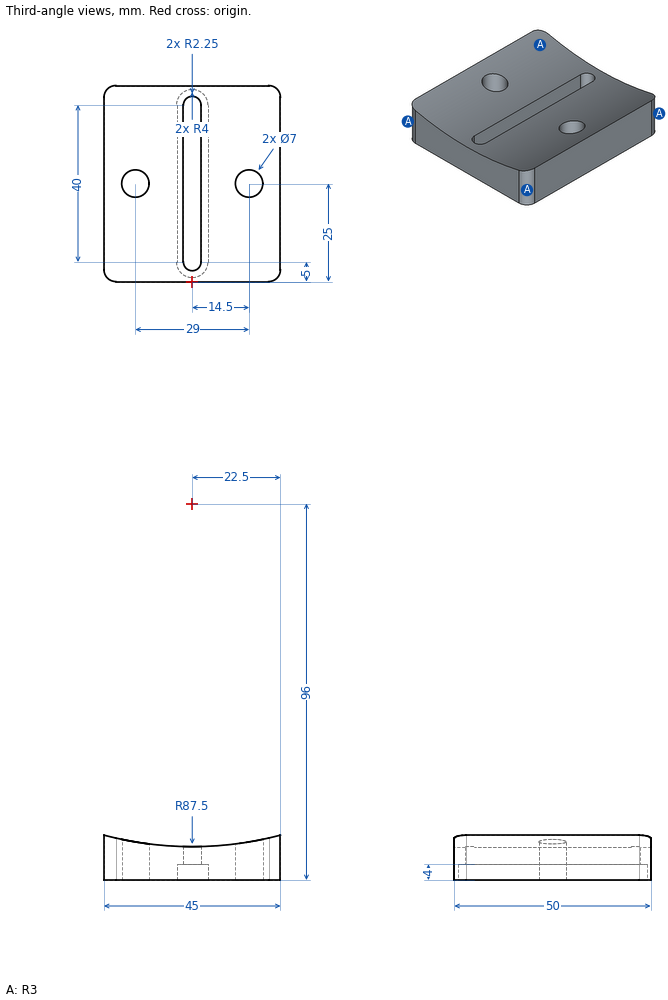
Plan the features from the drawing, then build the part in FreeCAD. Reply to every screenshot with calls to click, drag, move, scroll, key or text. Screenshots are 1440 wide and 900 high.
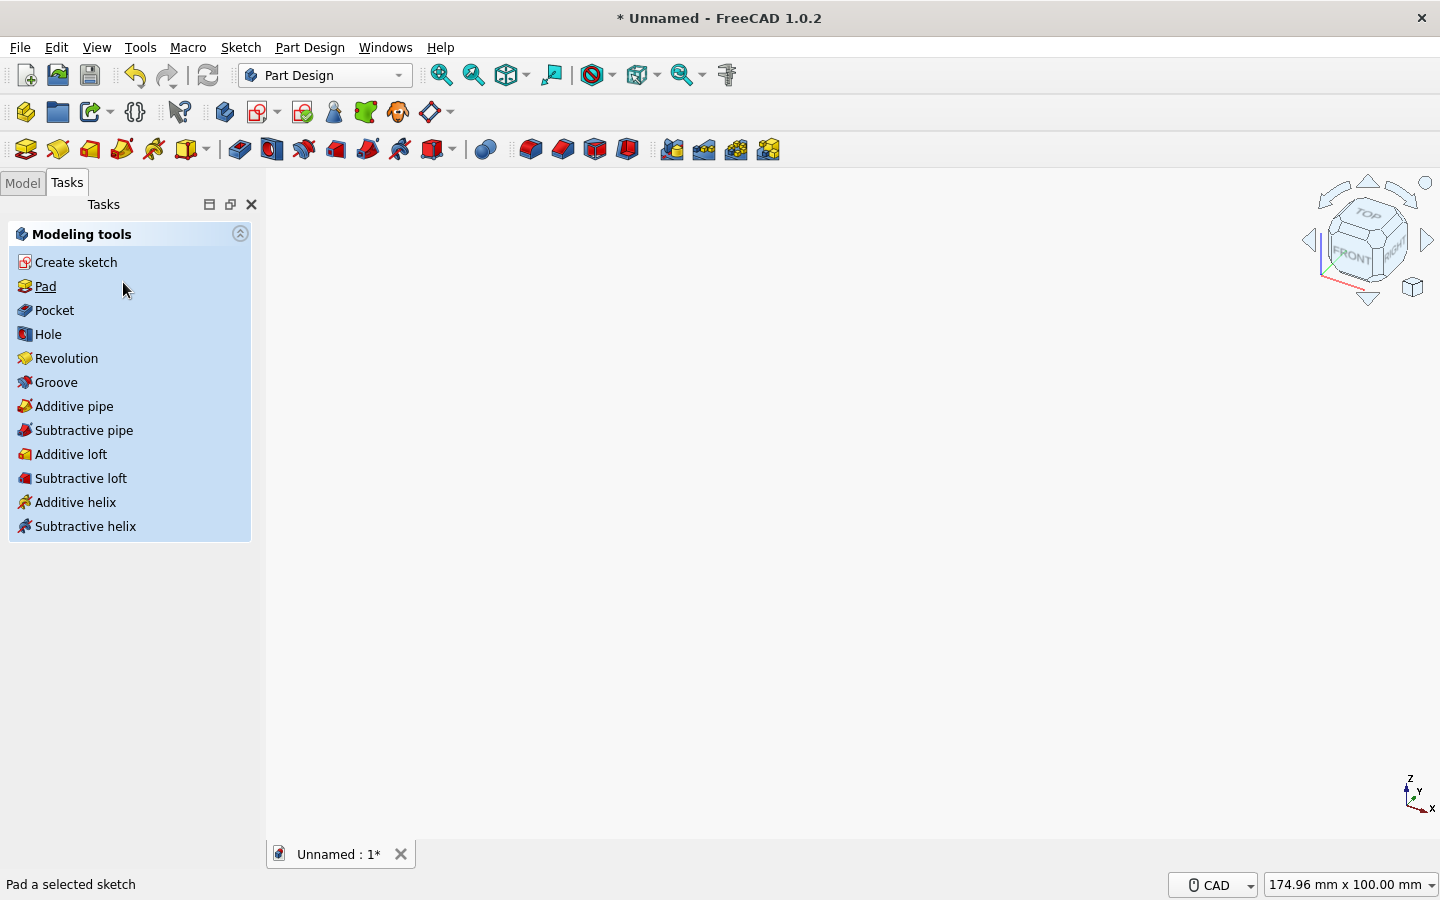
click(26, 150)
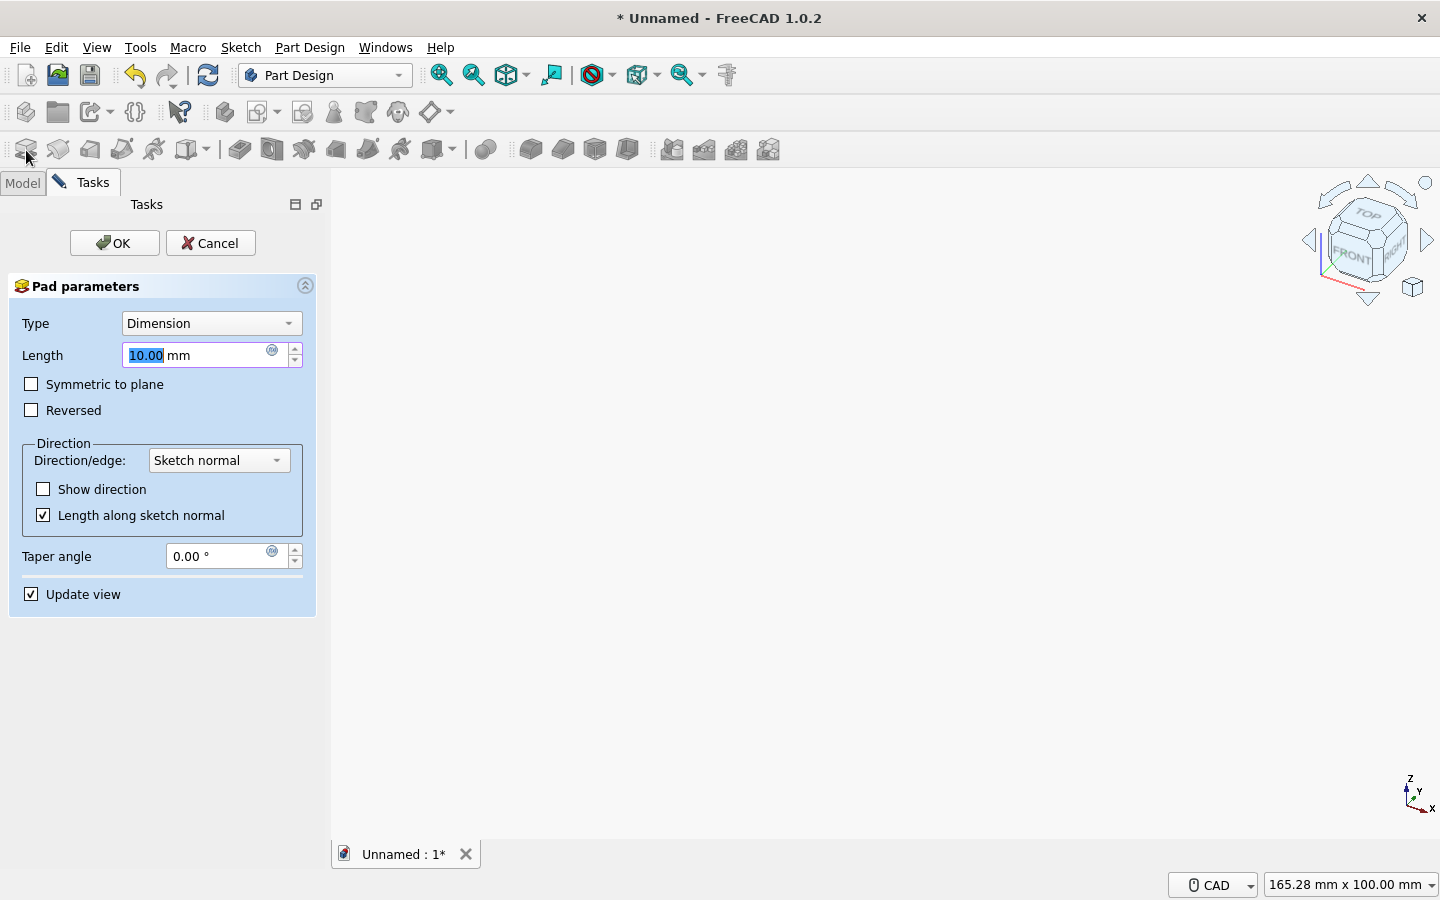
text(50)
key(Tab)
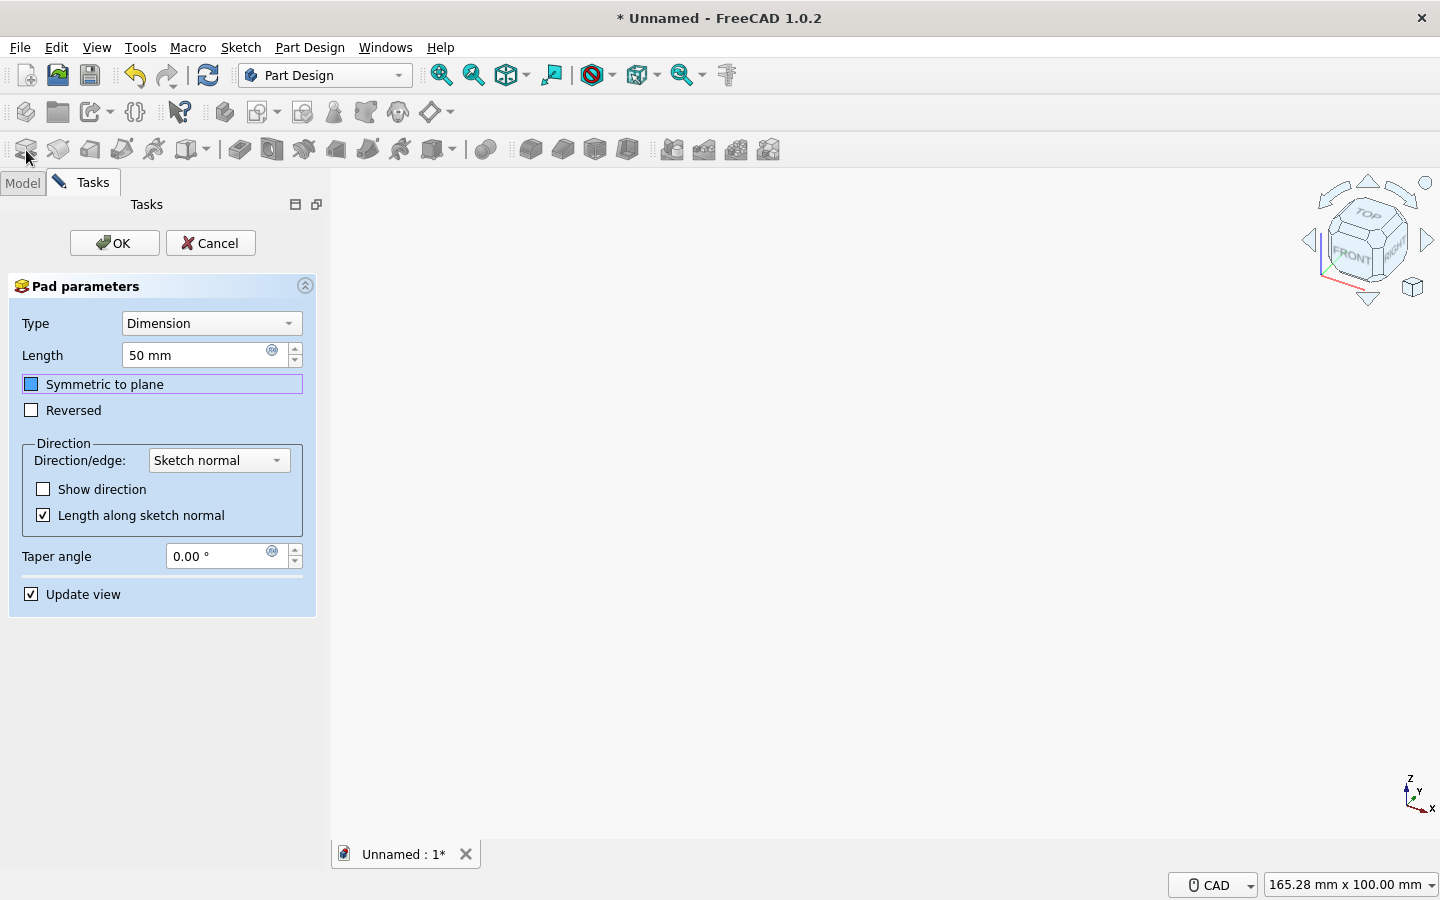
click(30, 410)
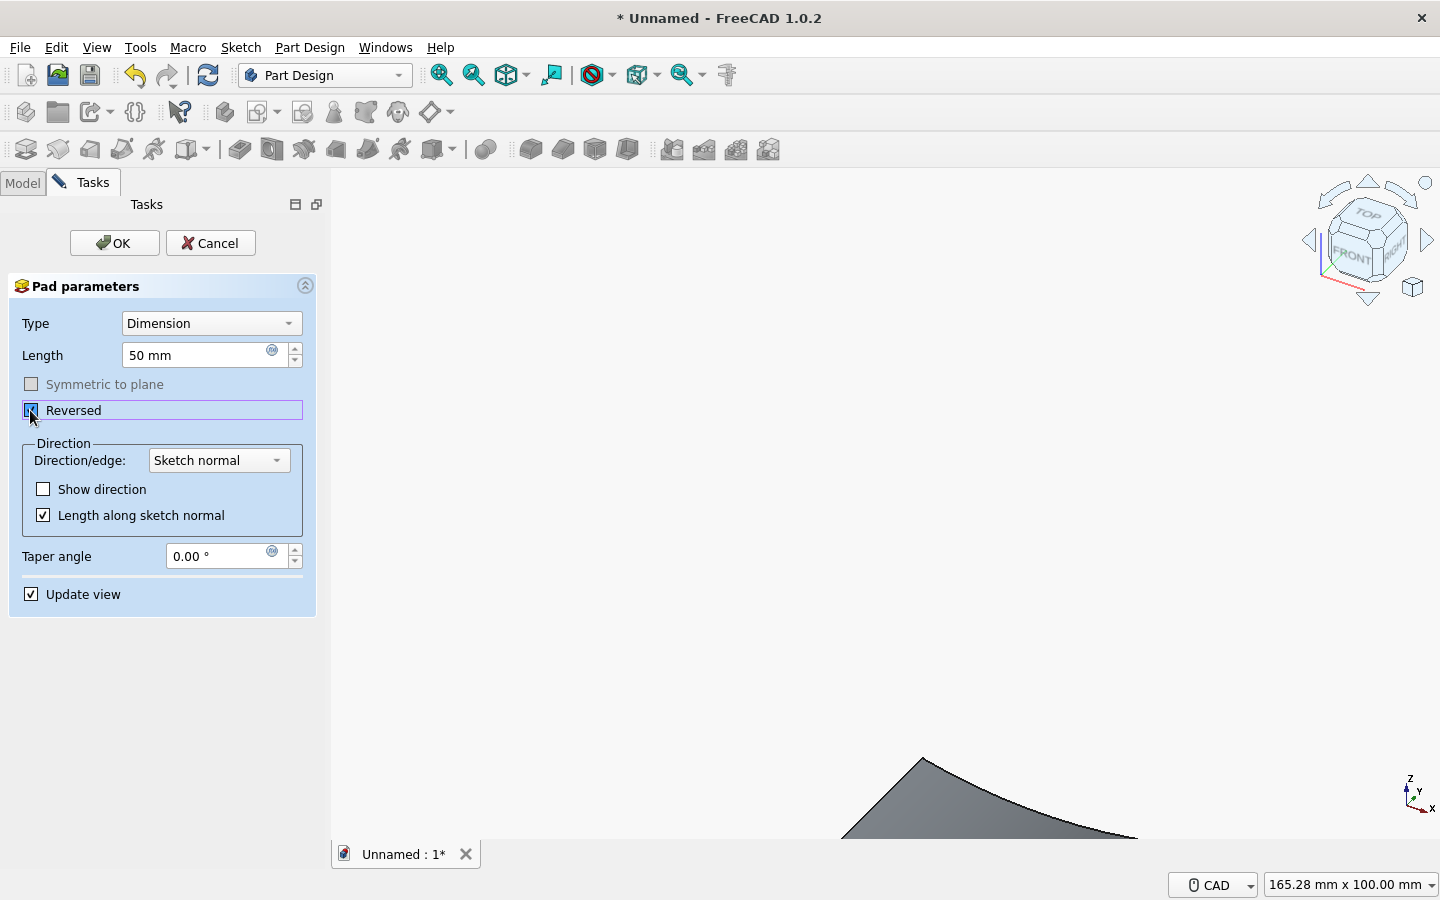
click(115, 243)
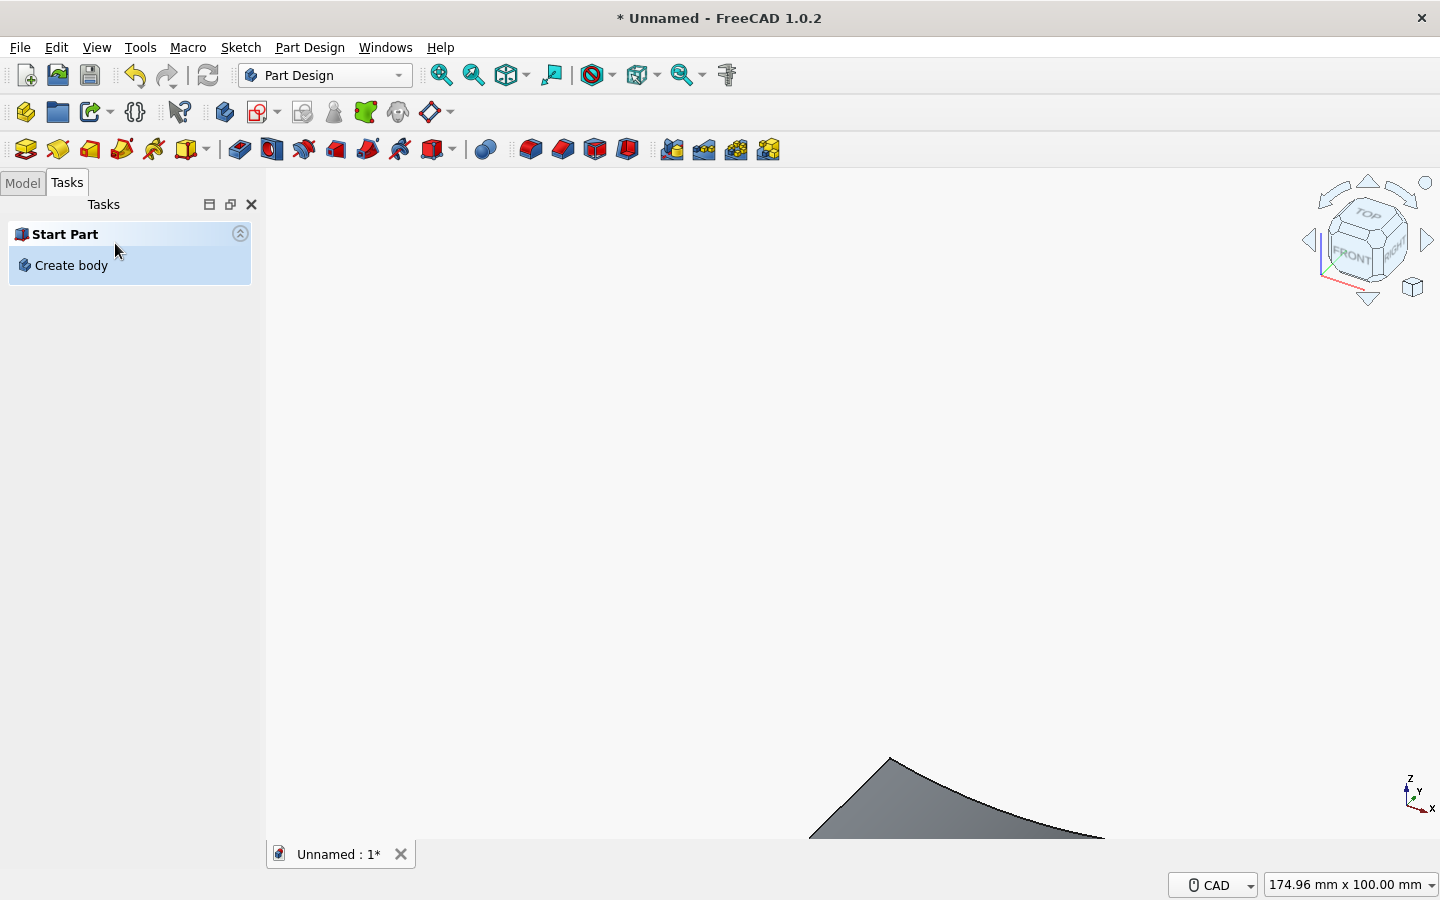
click(442, 76)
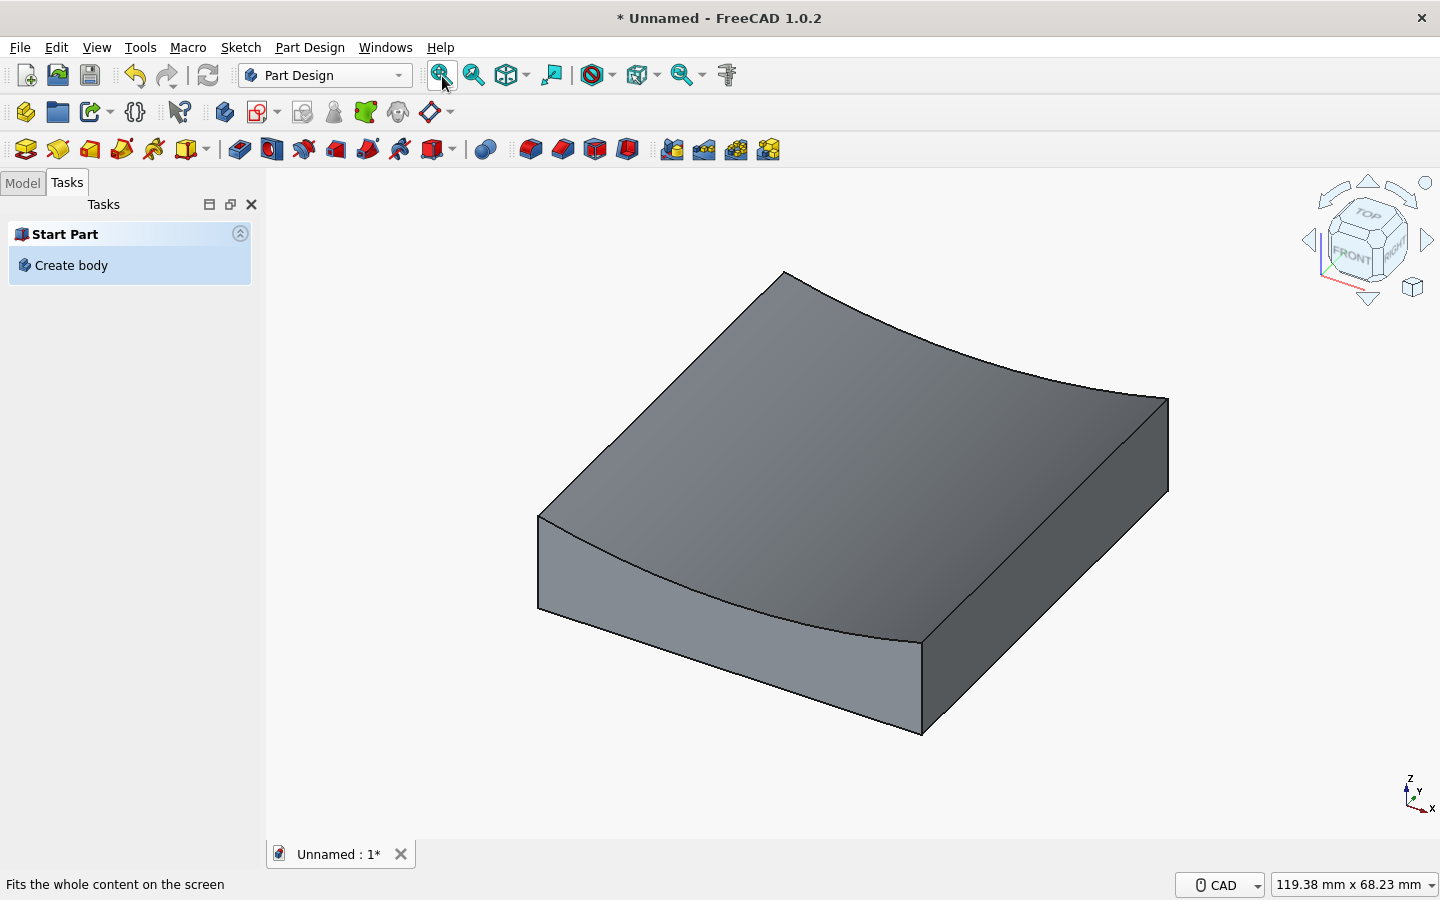
key(5)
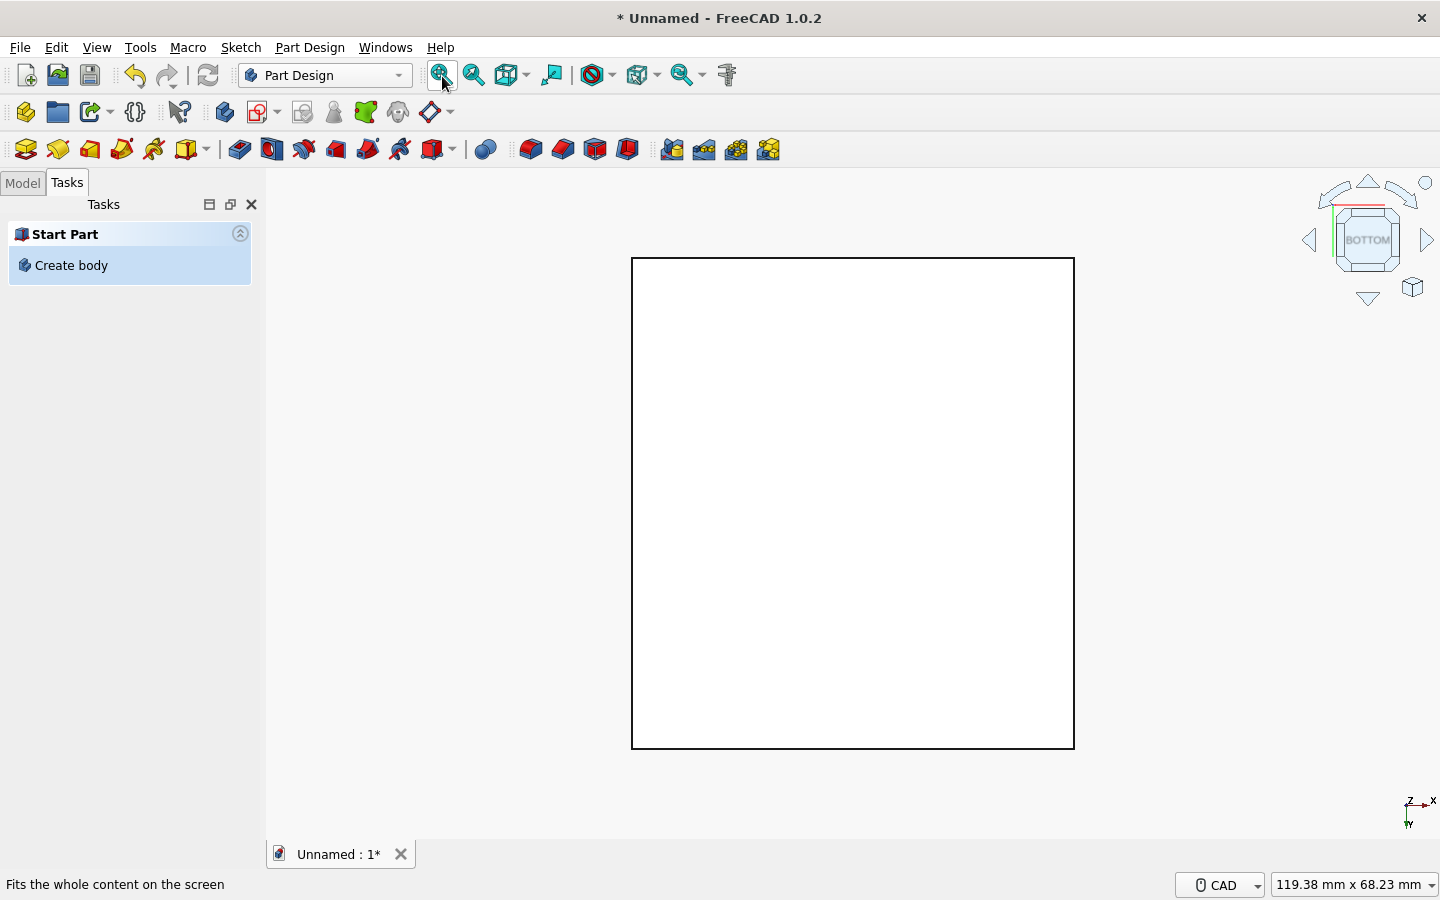
click(853, 502)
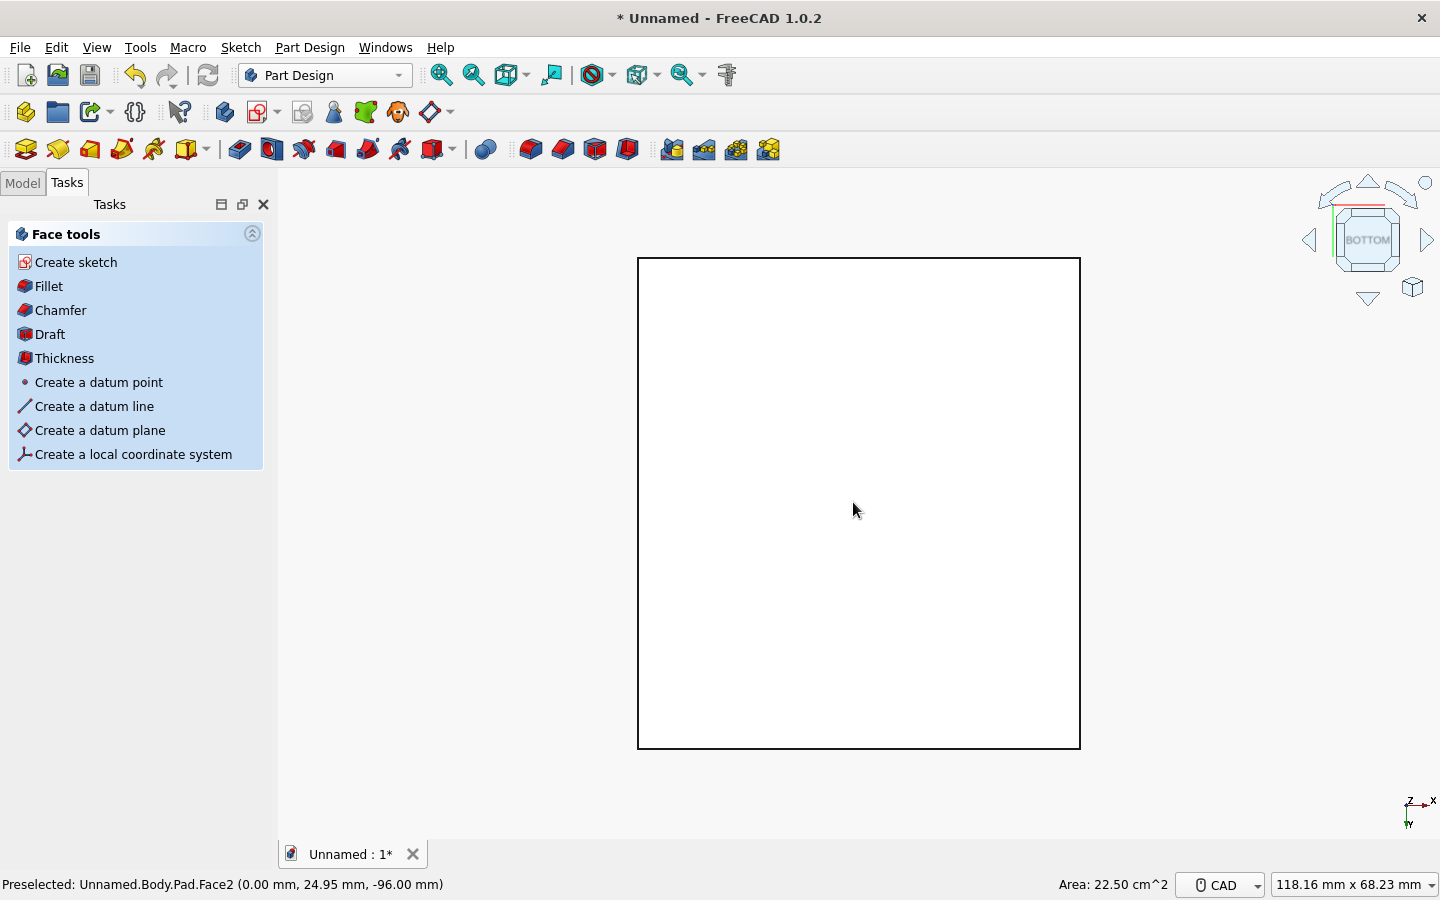
click(258, 112)